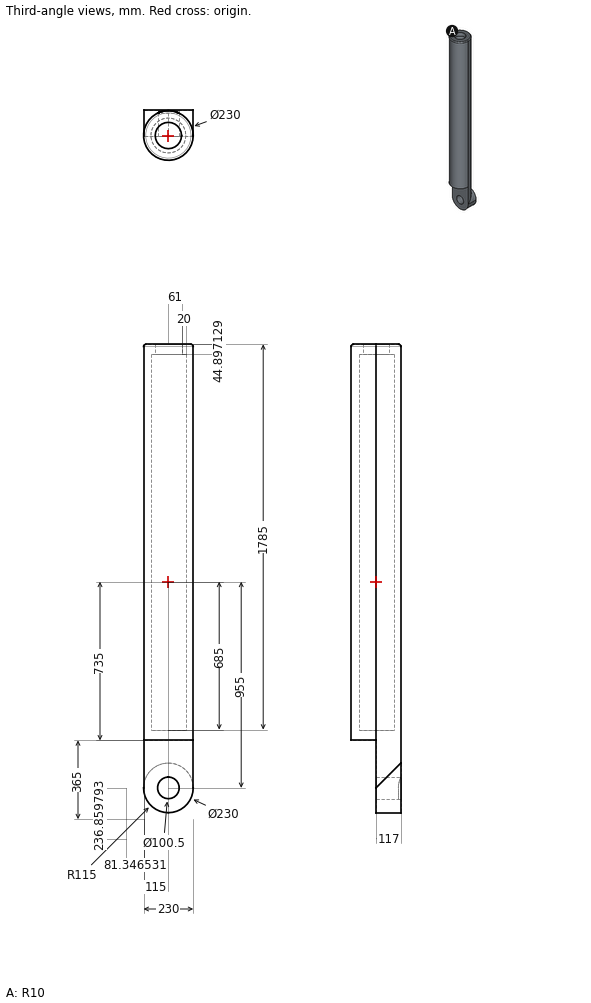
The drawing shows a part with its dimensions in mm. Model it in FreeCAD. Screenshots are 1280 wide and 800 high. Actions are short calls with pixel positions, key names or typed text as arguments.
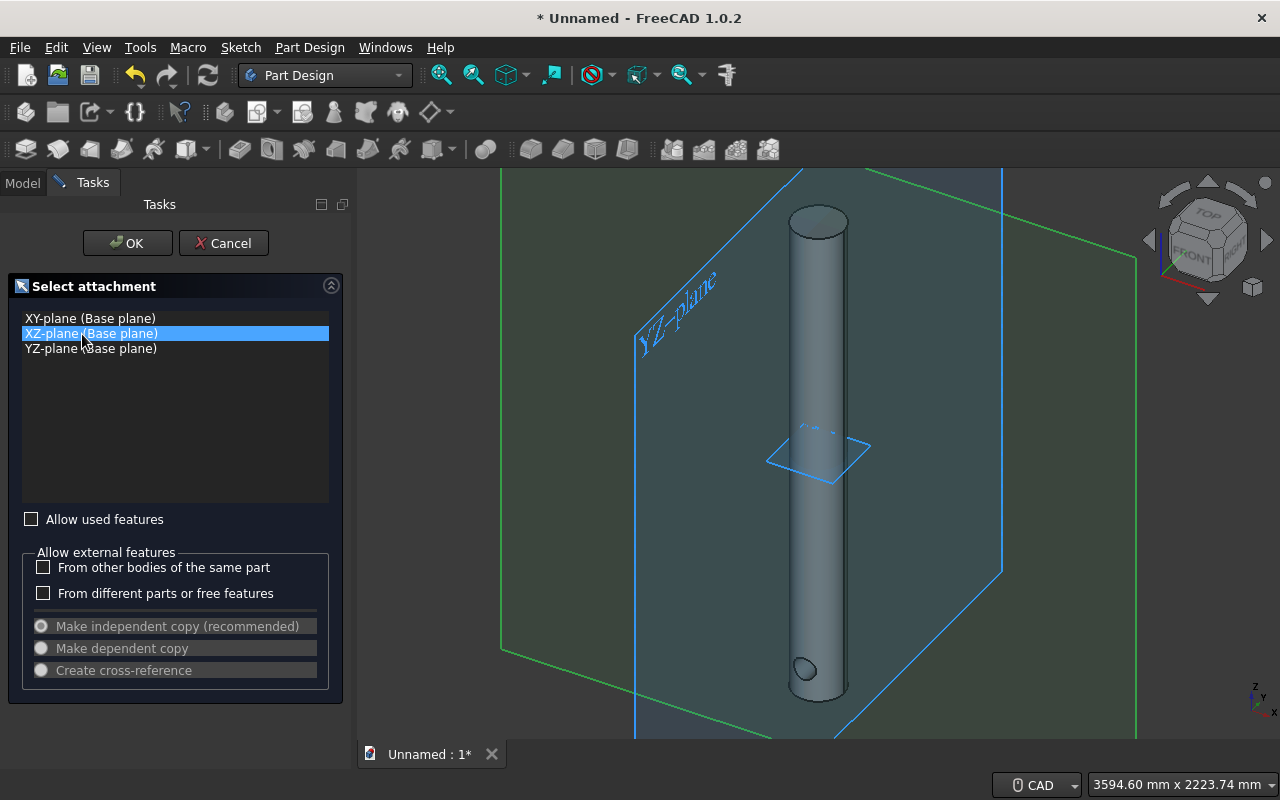
click(128, 243)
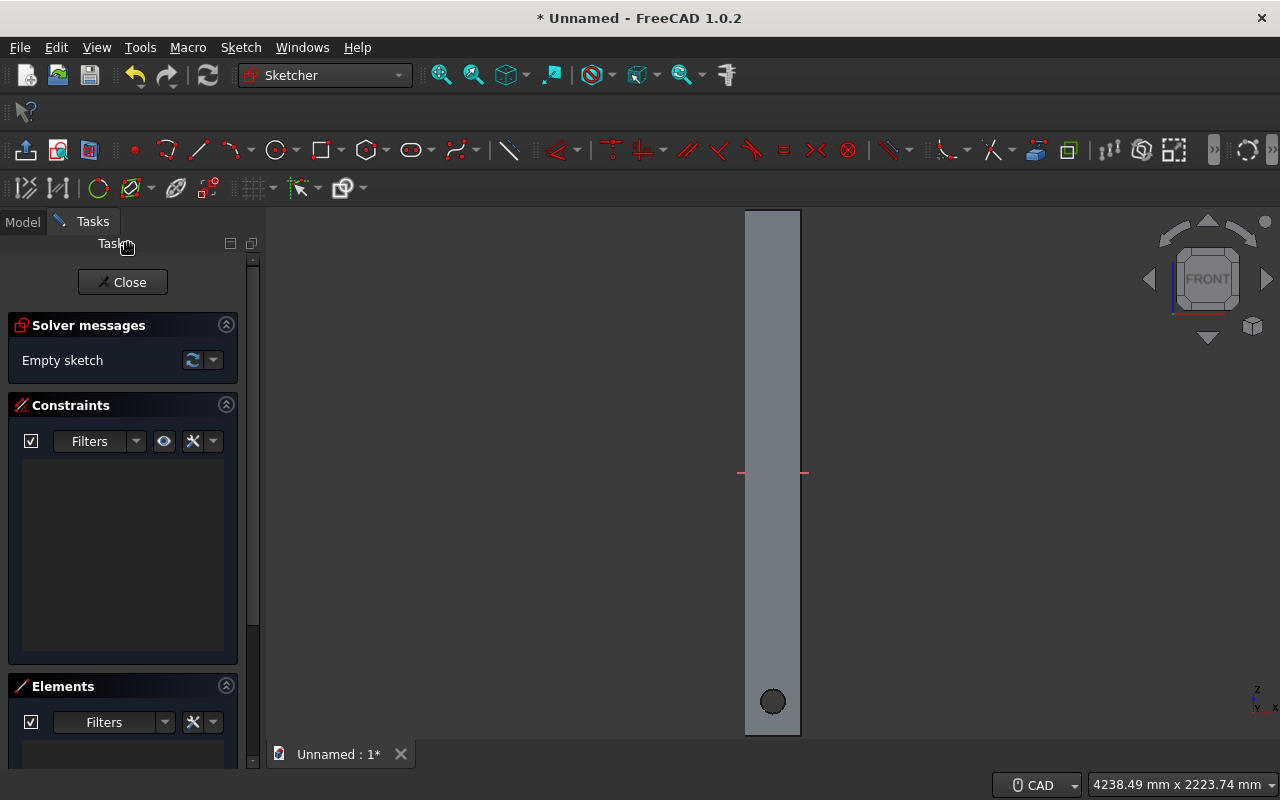
click(90, 150)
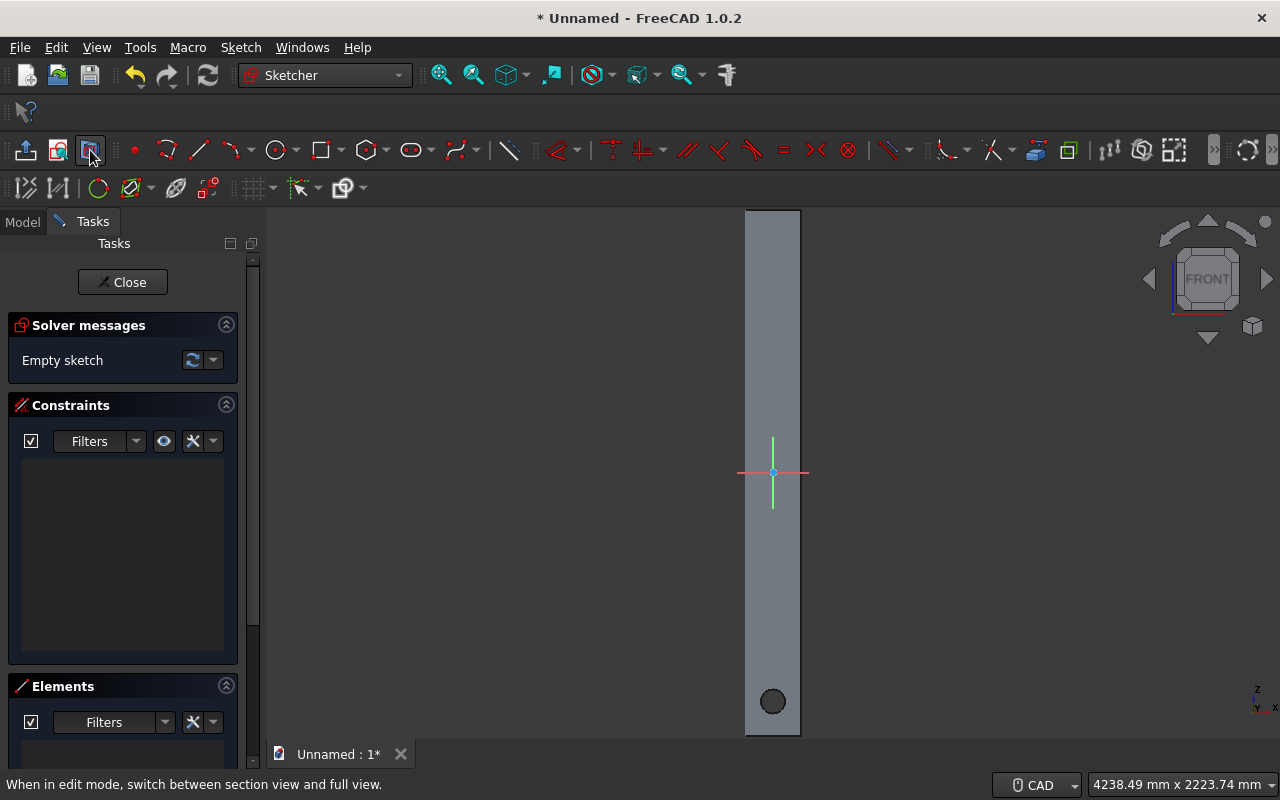
scroll(704, 473, down, 5)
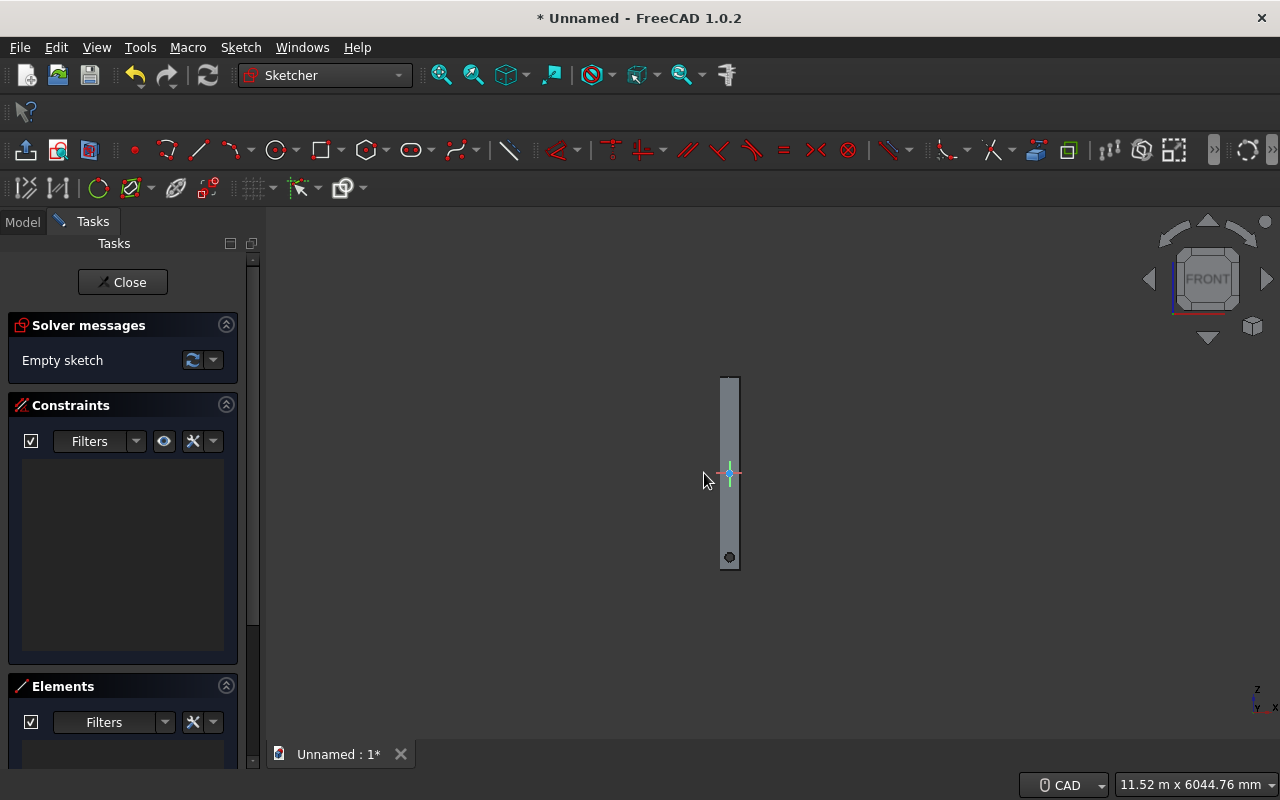
scroll(732, 562, up, 12)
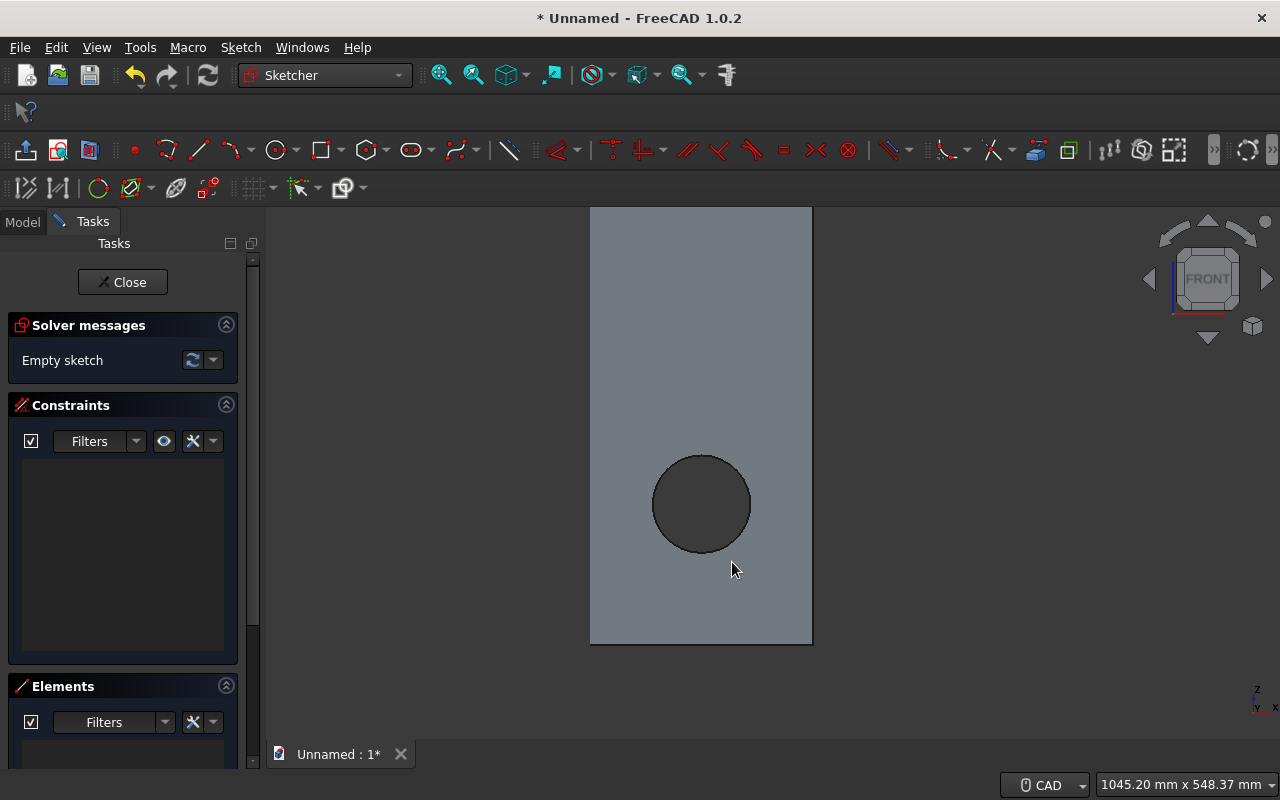
click(322, 150)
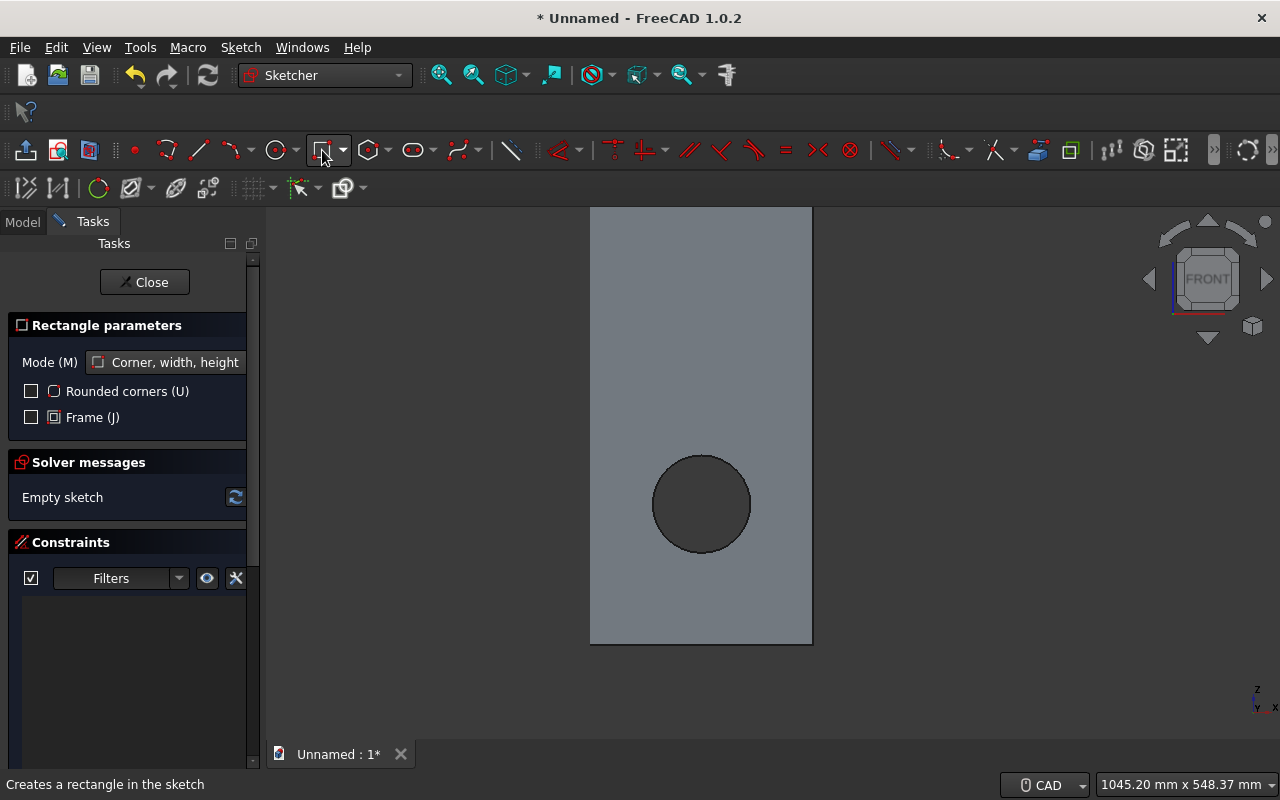
click(590, 291)
click(813, 645)
key(Escape)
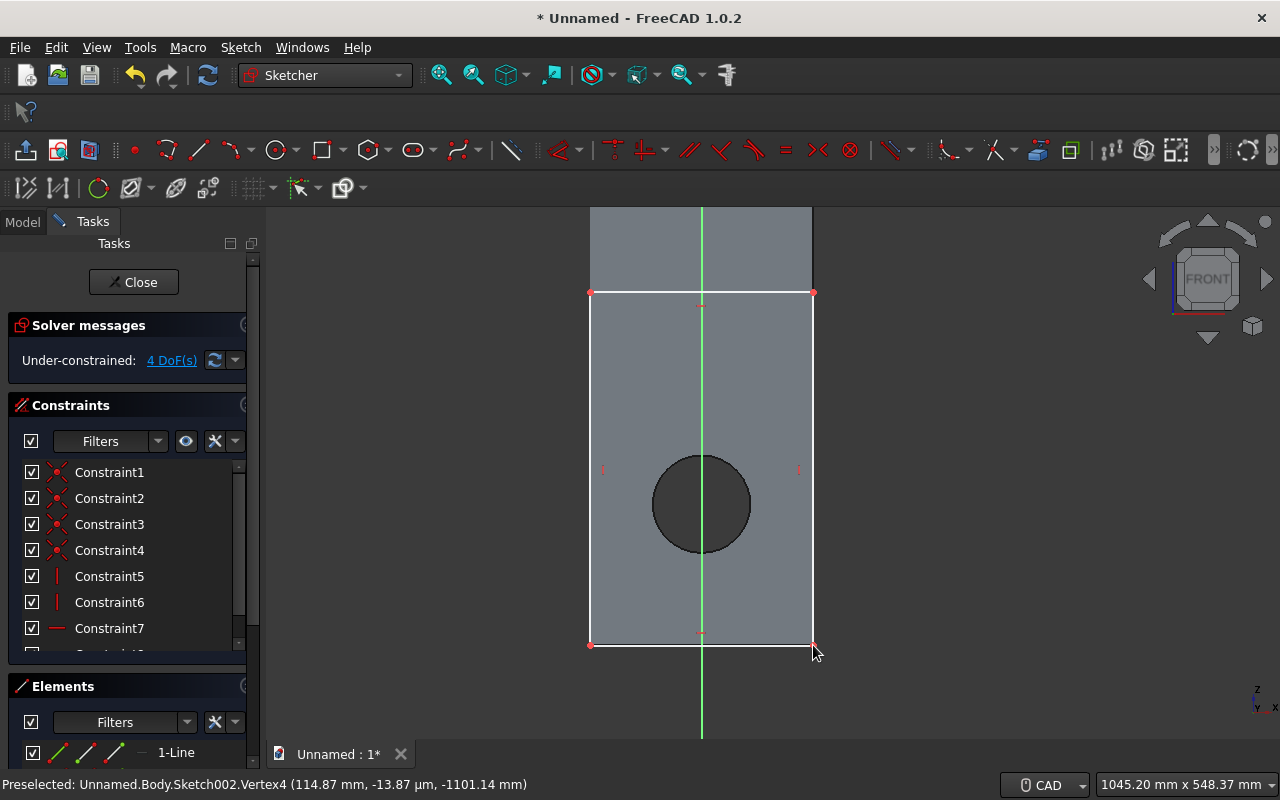
key(d)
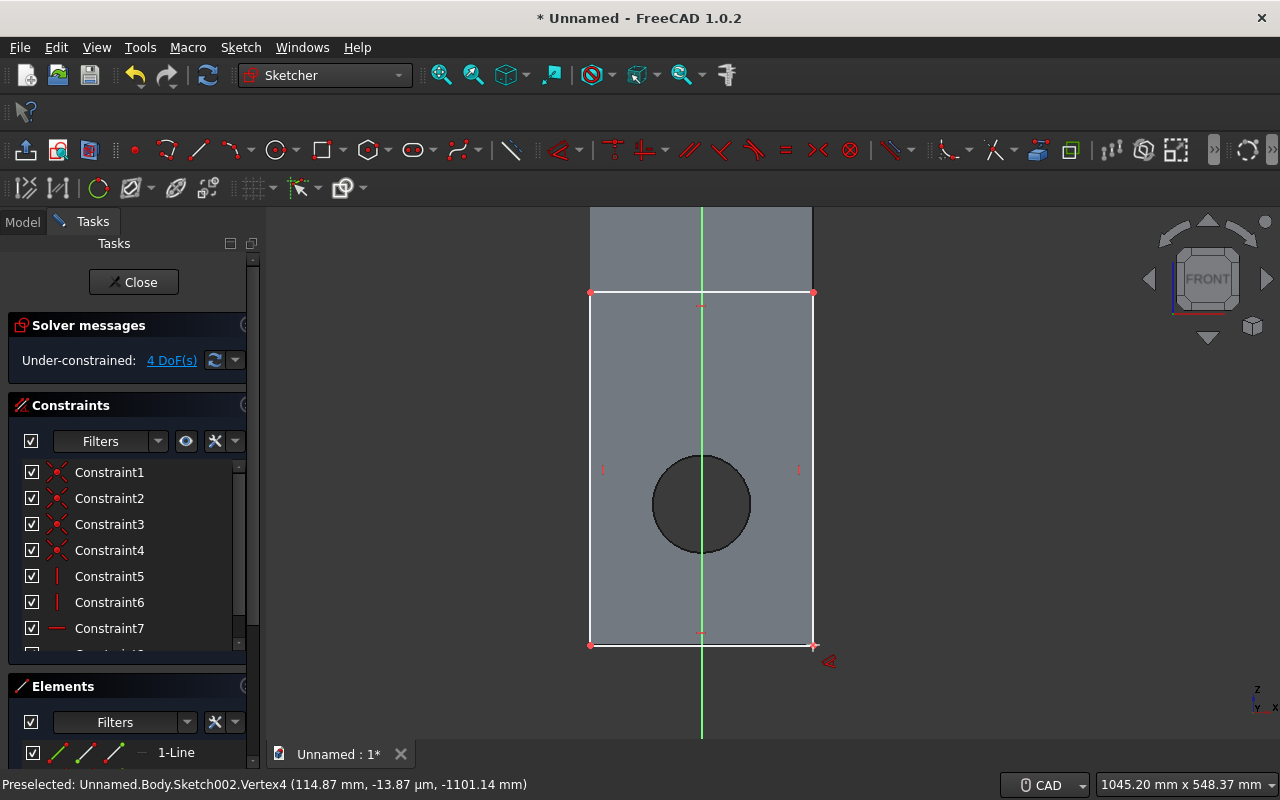
click(590, 398)
click(556, 469)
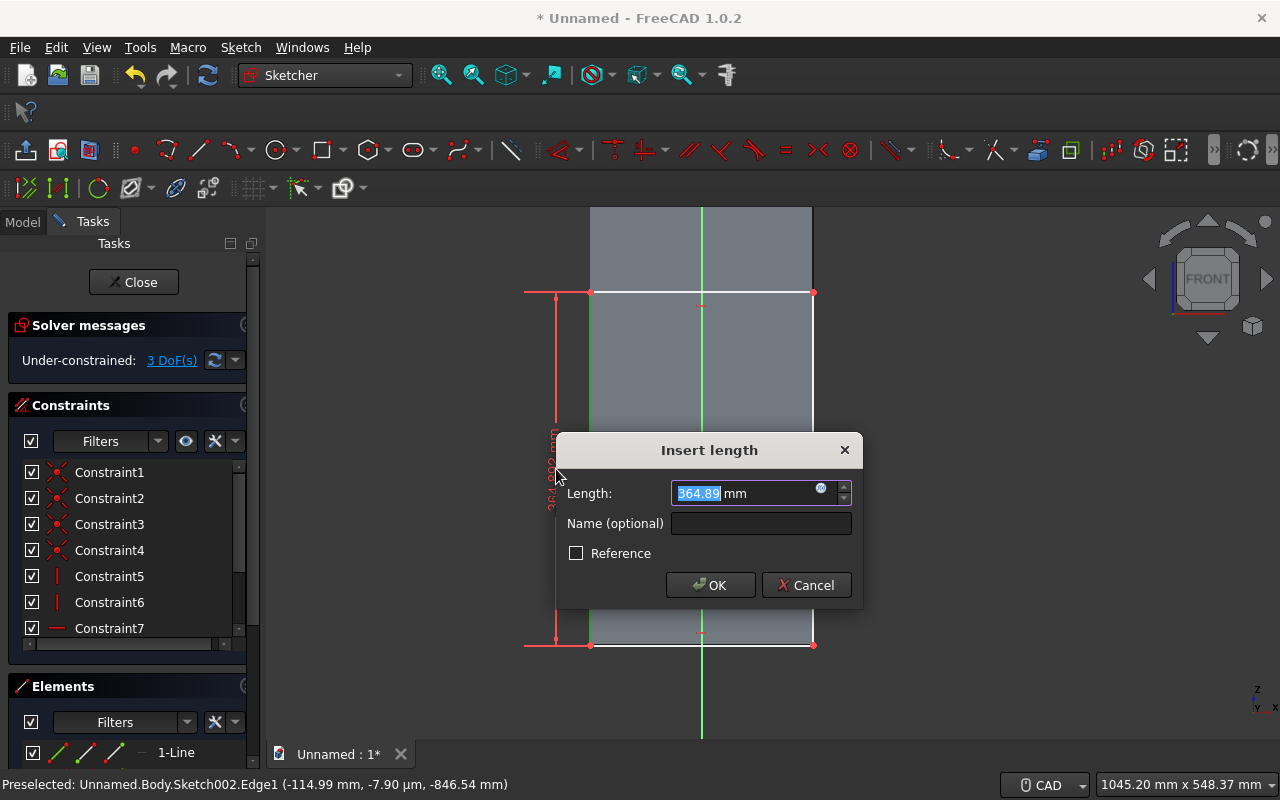
text(365)
key(Return)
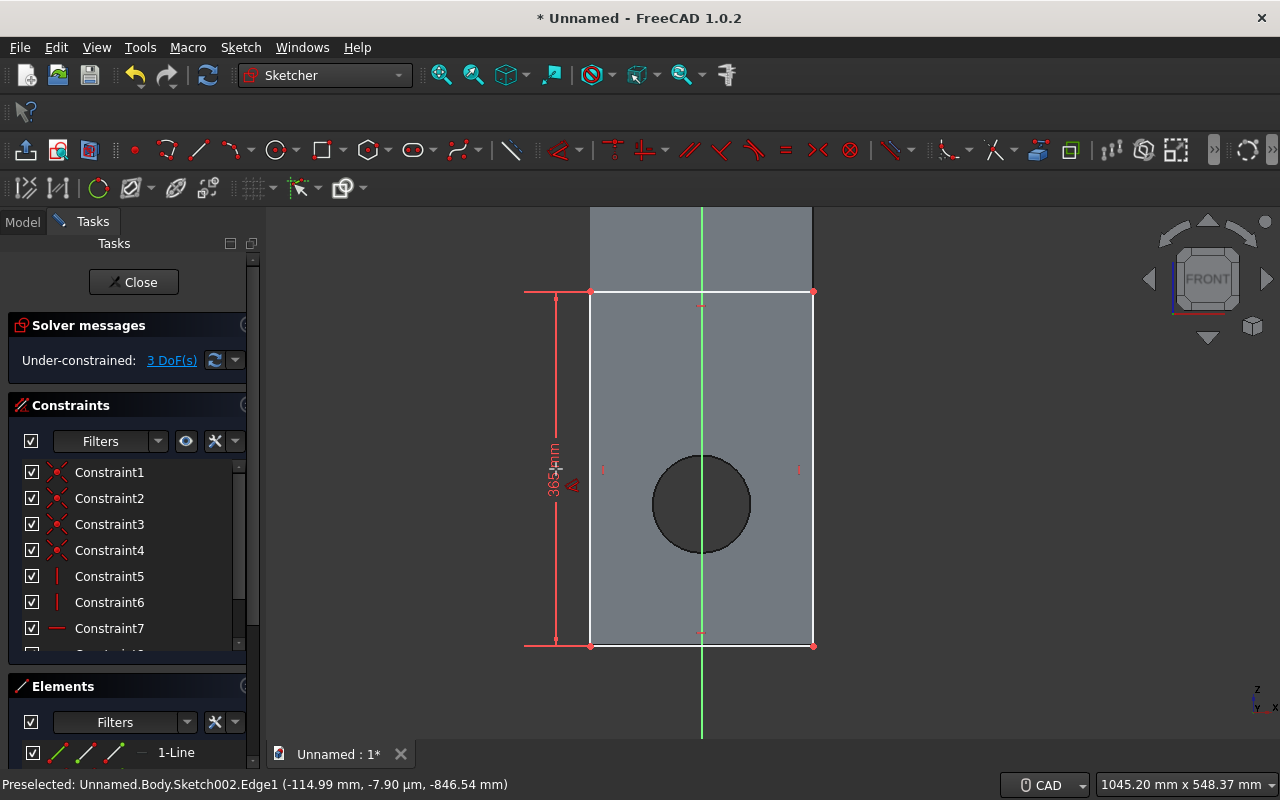
click(657, 646)
click(650, 680)